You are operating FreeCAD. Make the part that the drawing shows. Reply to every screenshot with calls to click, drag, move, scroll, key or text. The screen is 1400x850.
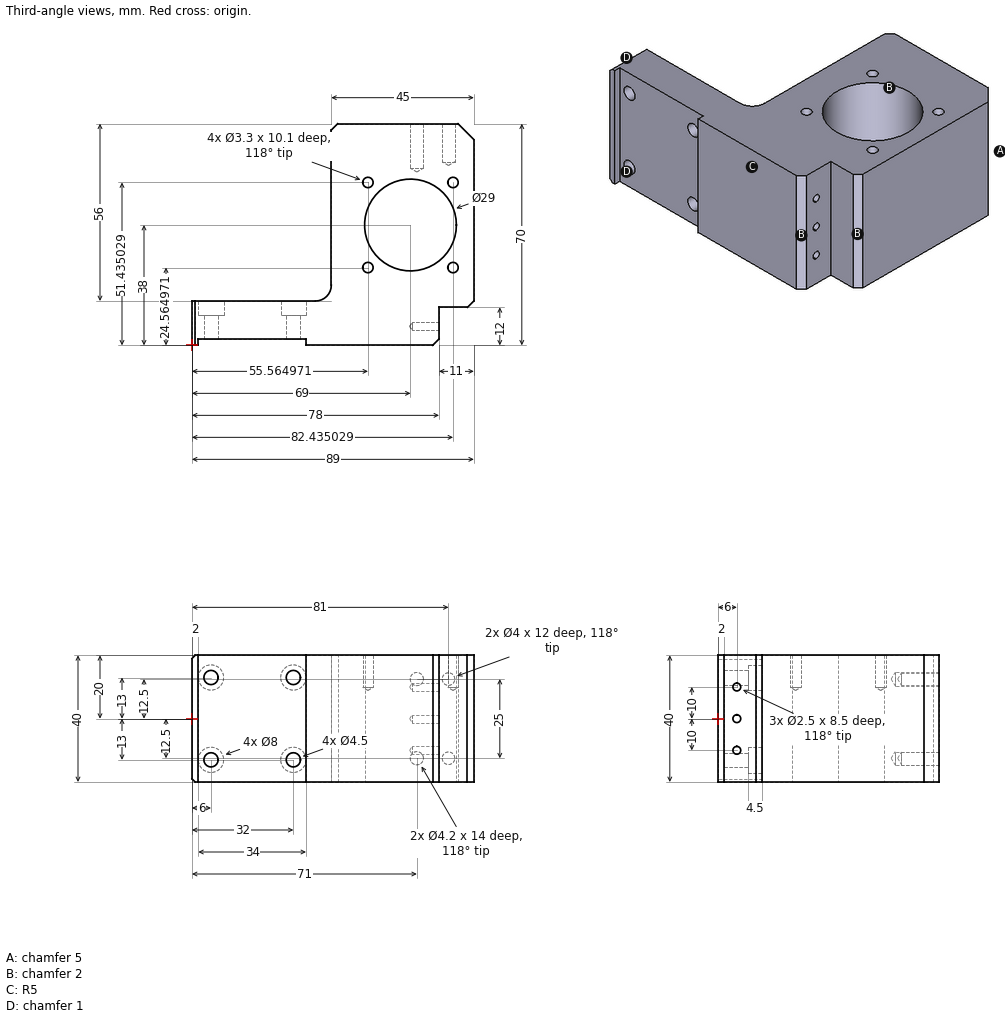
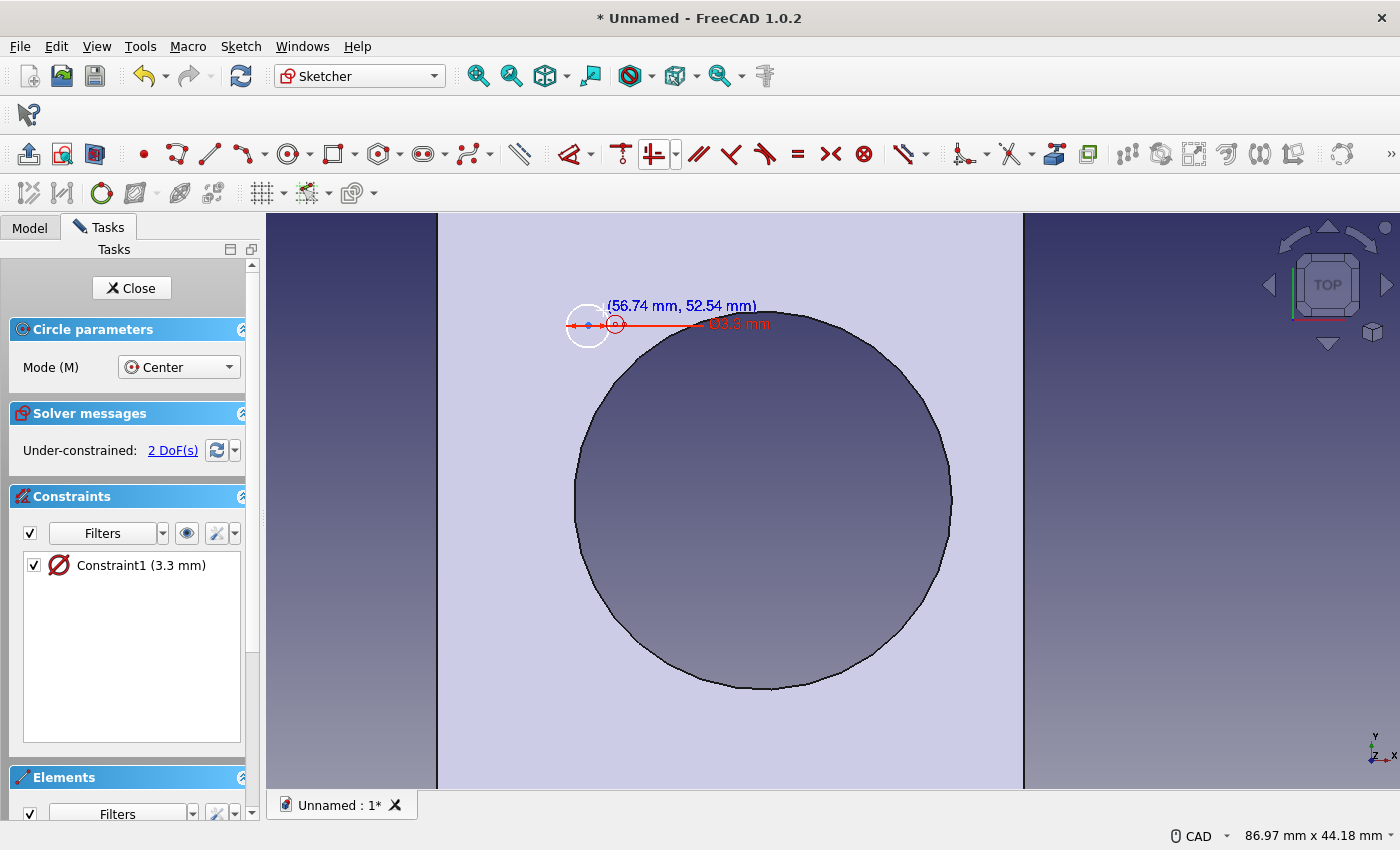
click(938, 325)
move(953, 310)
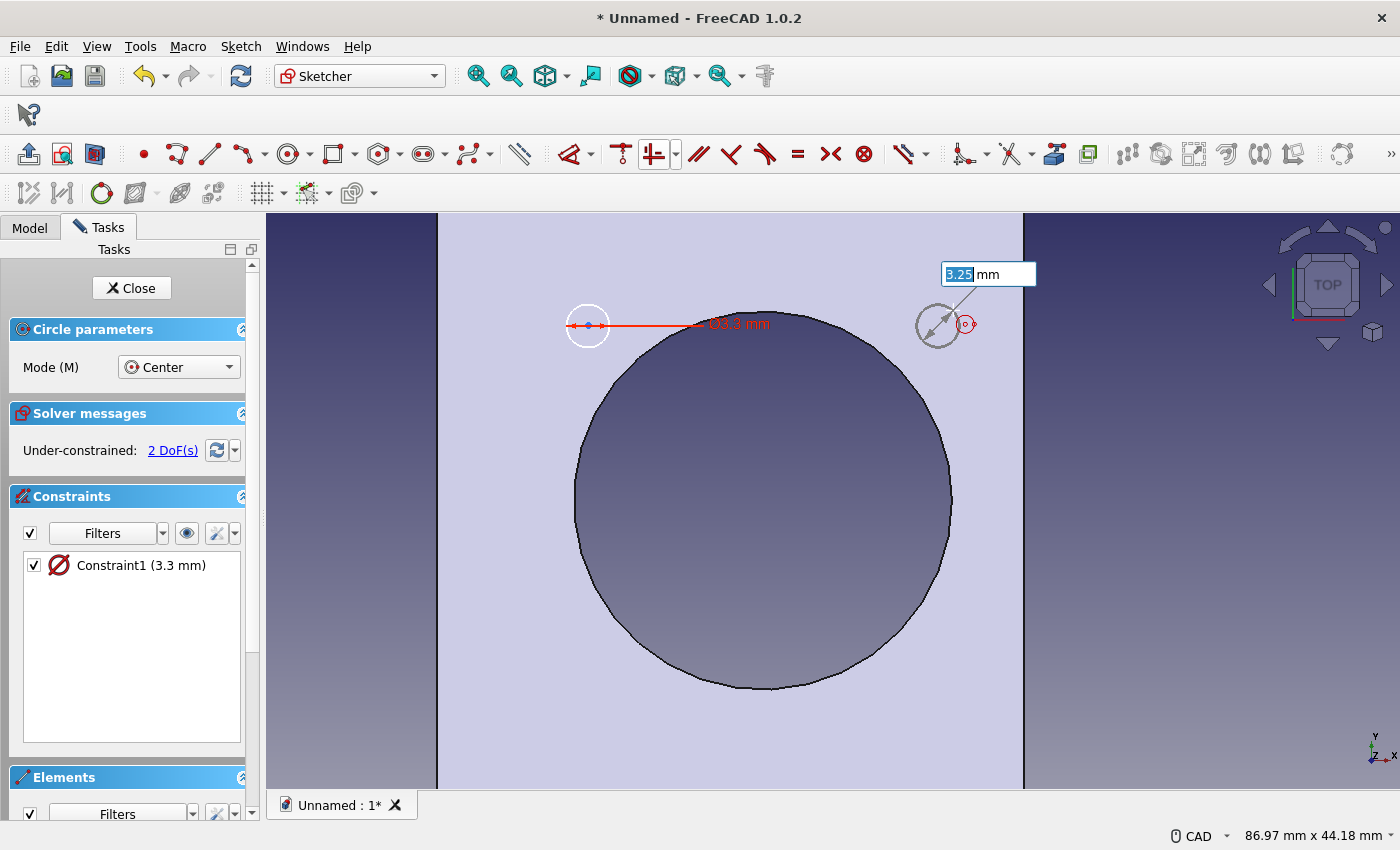
text(3.3)
key(Return)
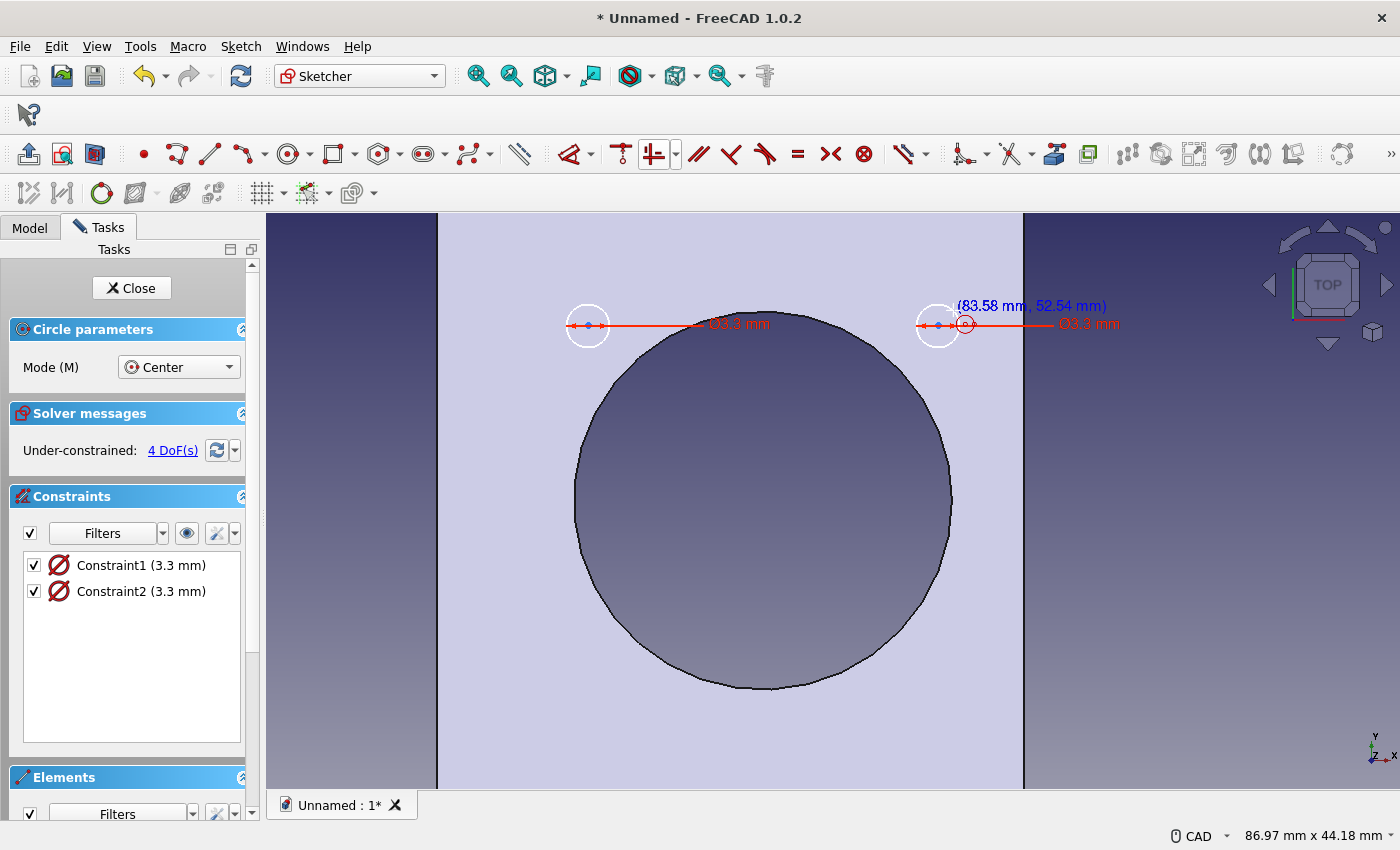
click(588, 676)
move(603, 661)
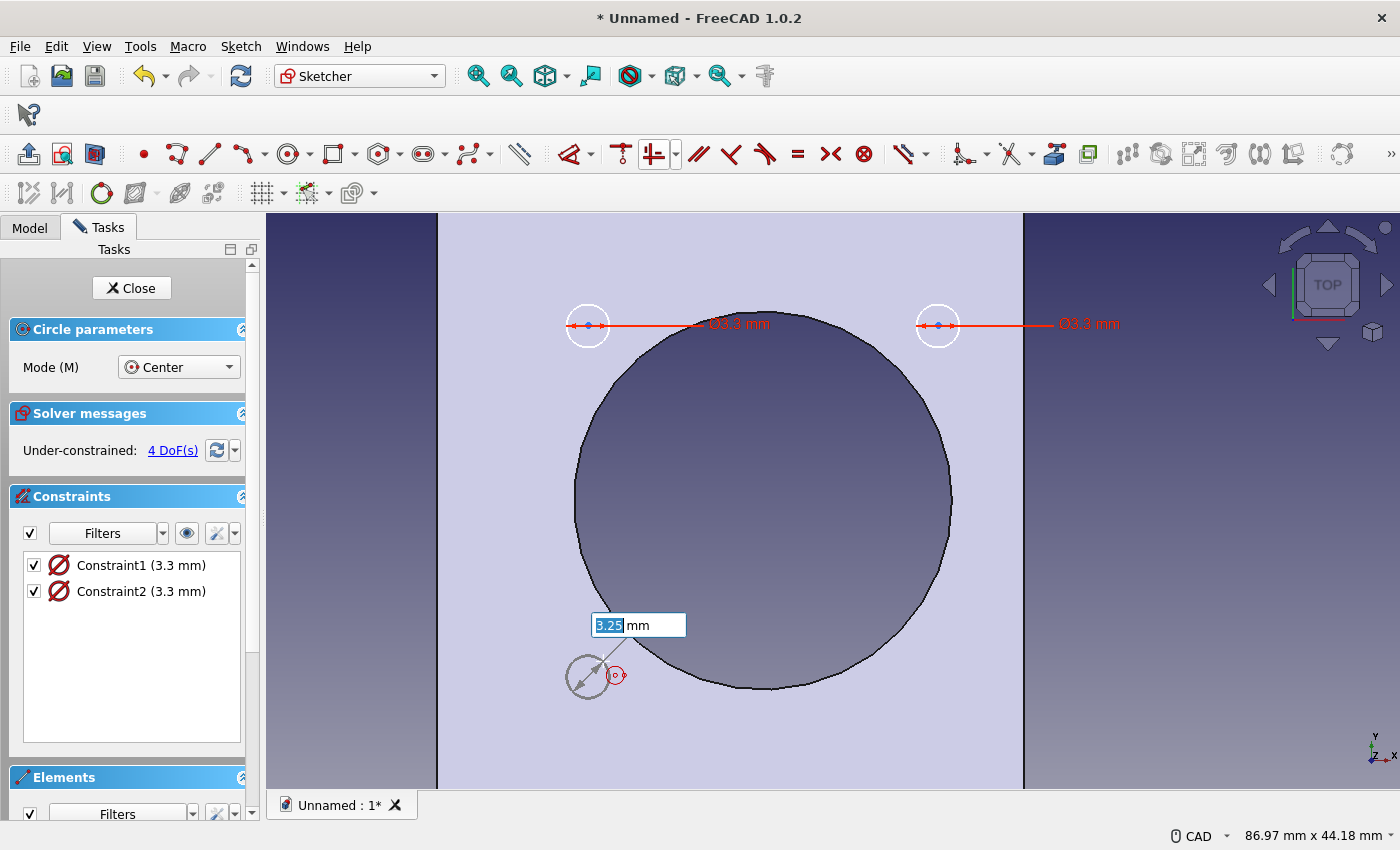
text(3.3)
key(Return)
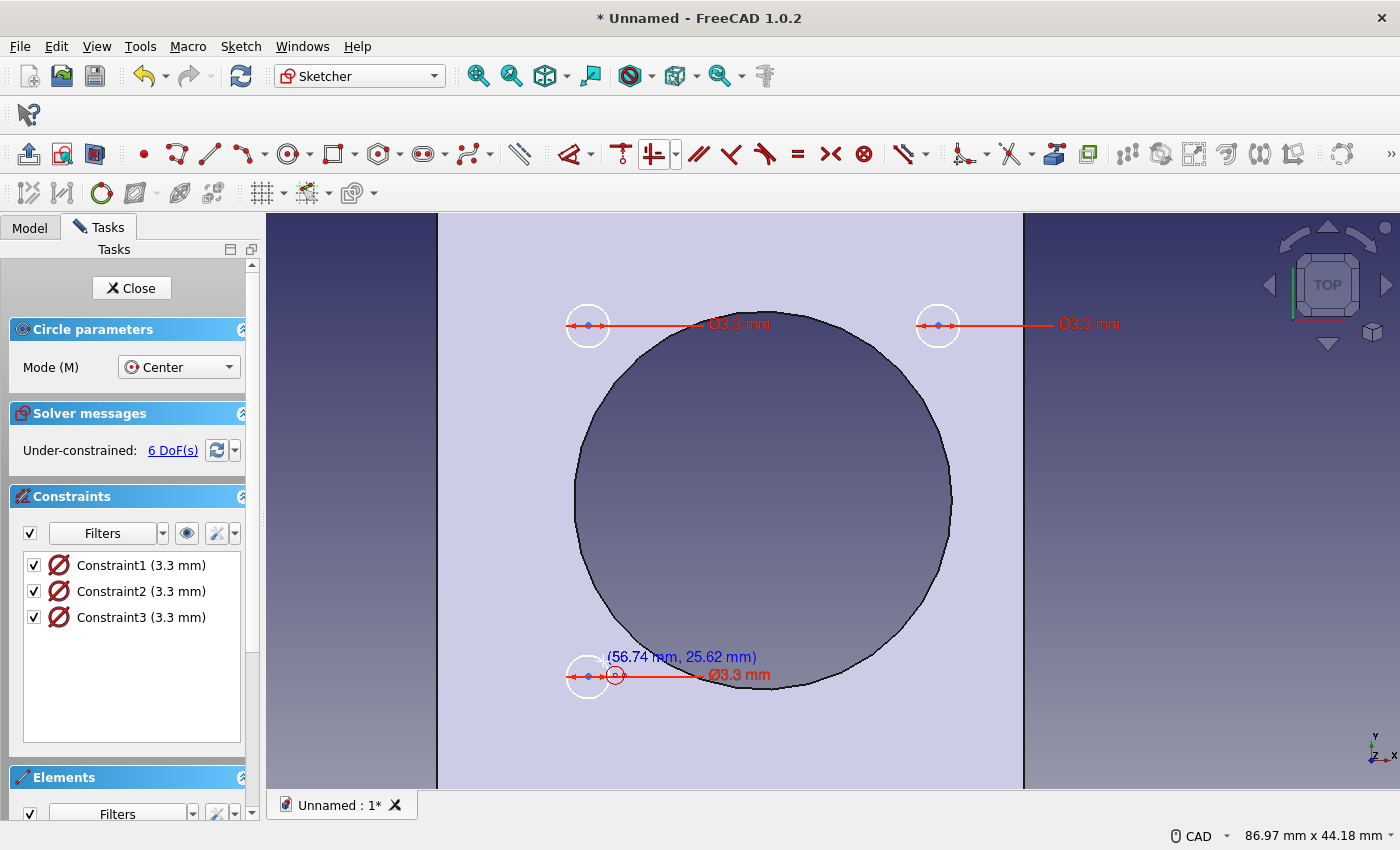
click(938, 676)
move(953, 661)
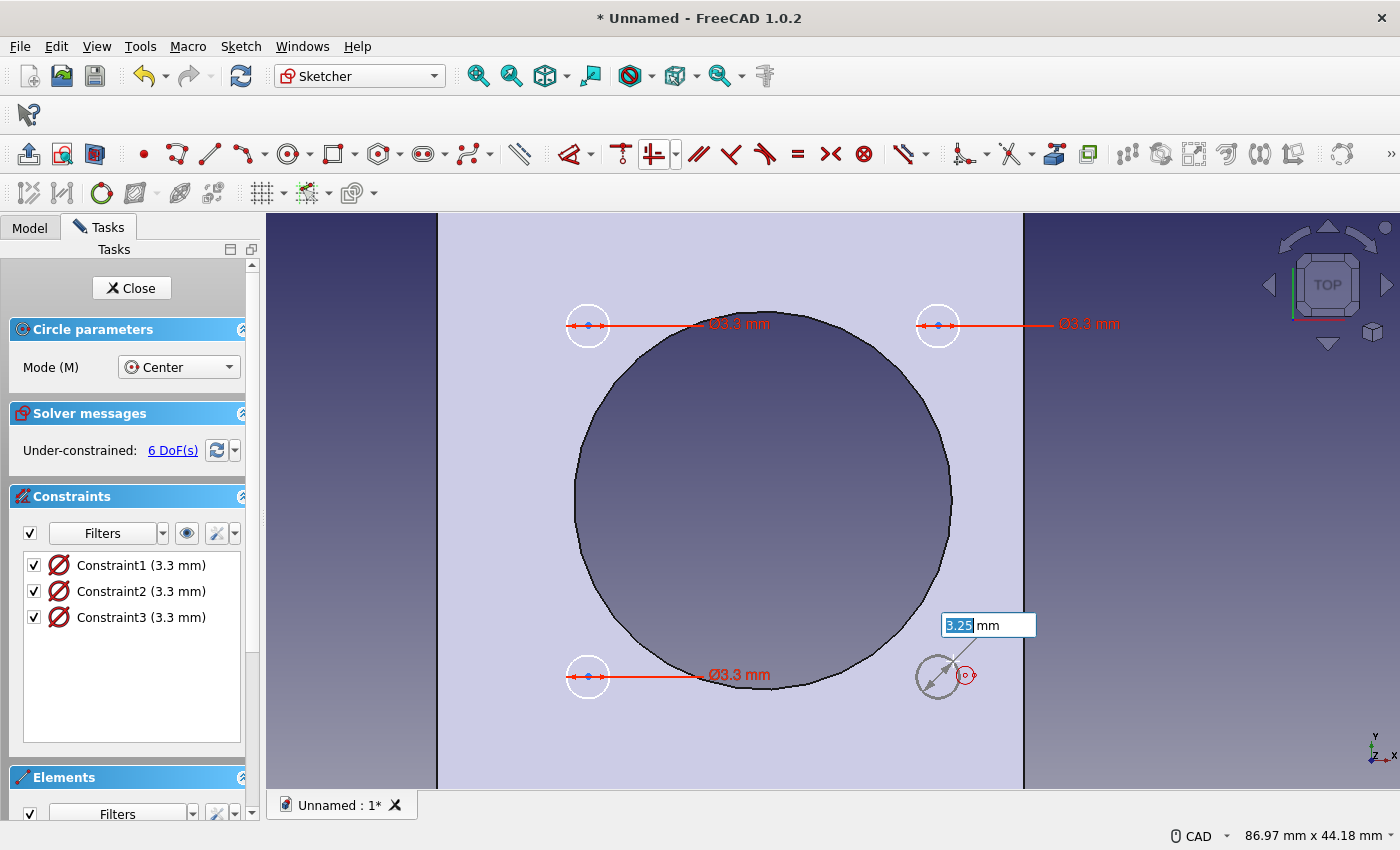
text(3.3)
key(Return)
key(Escape)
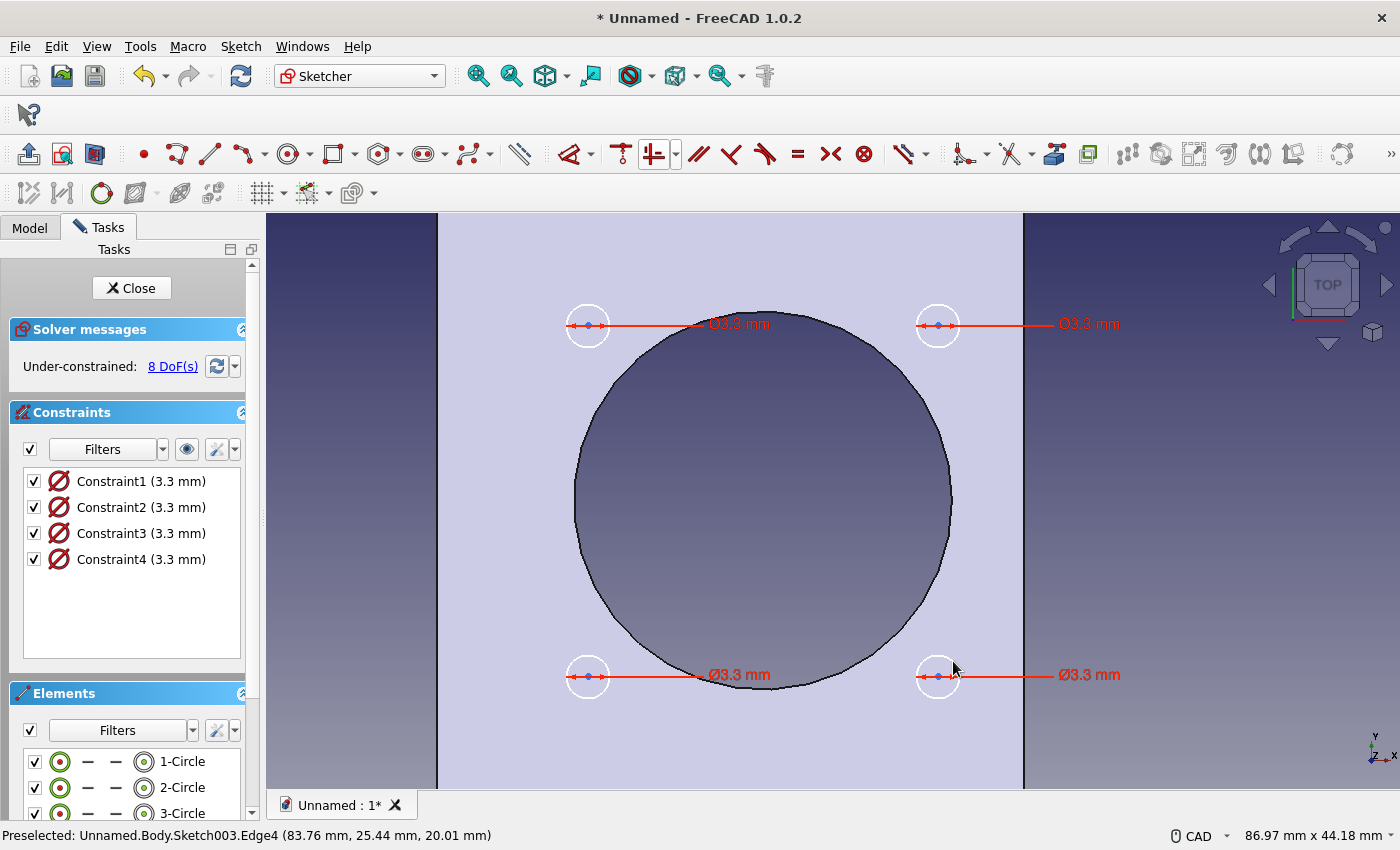
click(588, 326)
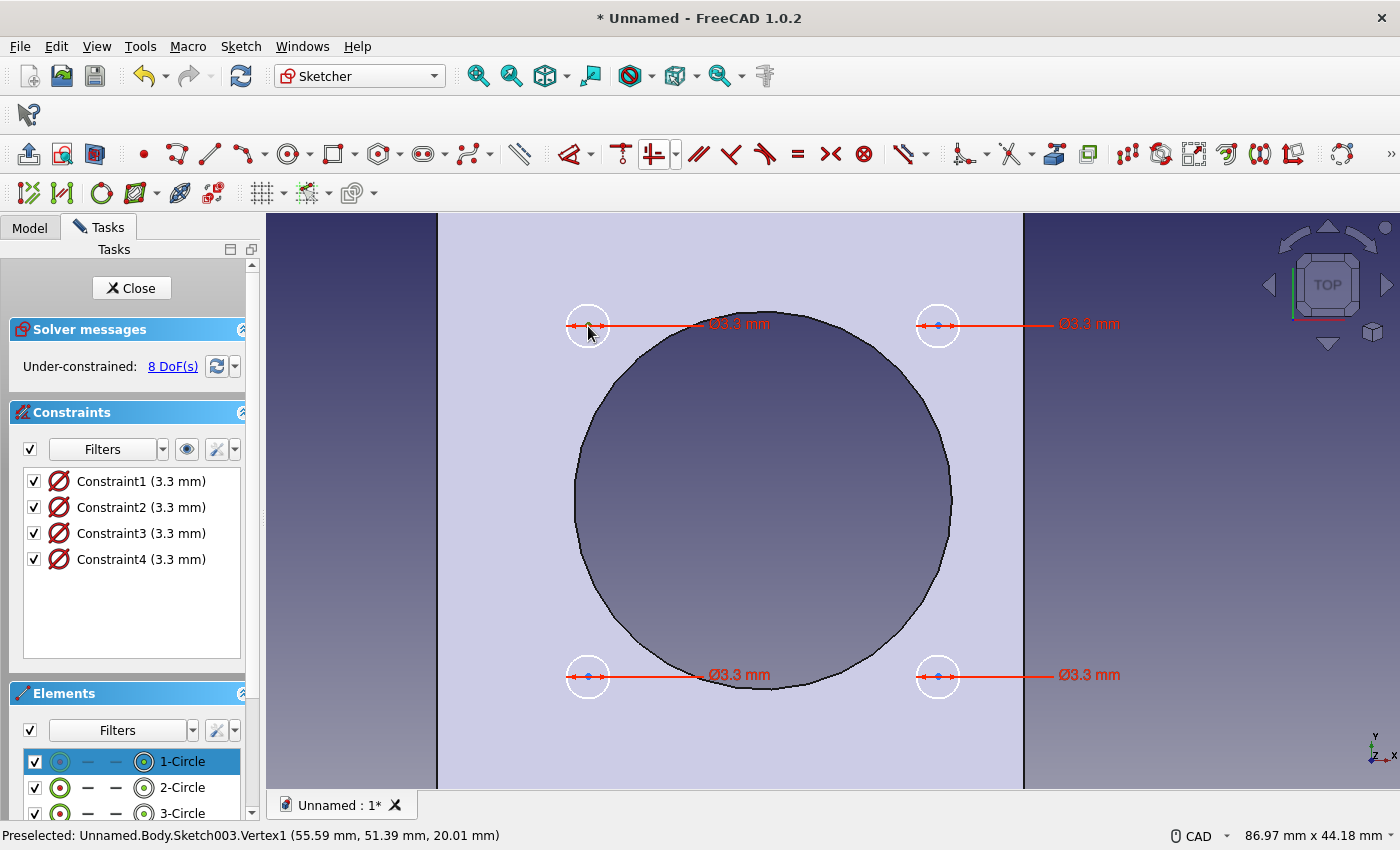
click(938, 326)